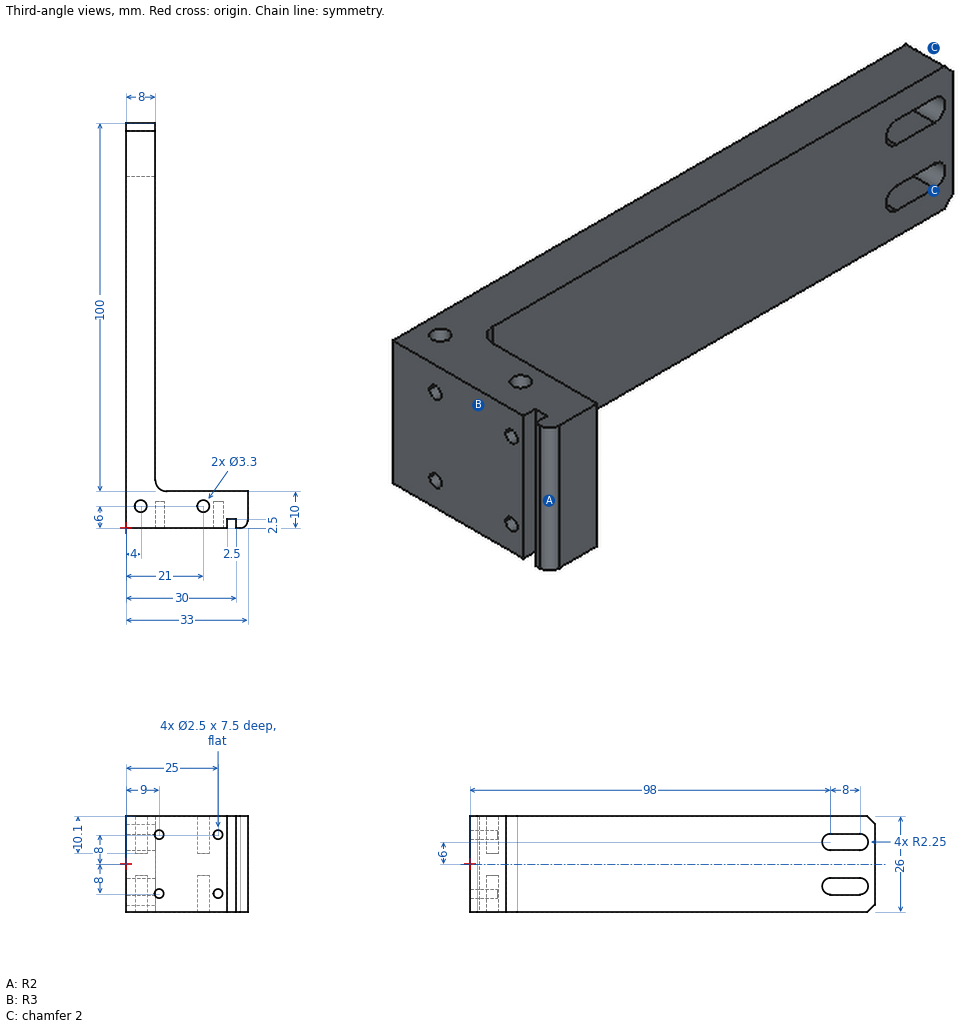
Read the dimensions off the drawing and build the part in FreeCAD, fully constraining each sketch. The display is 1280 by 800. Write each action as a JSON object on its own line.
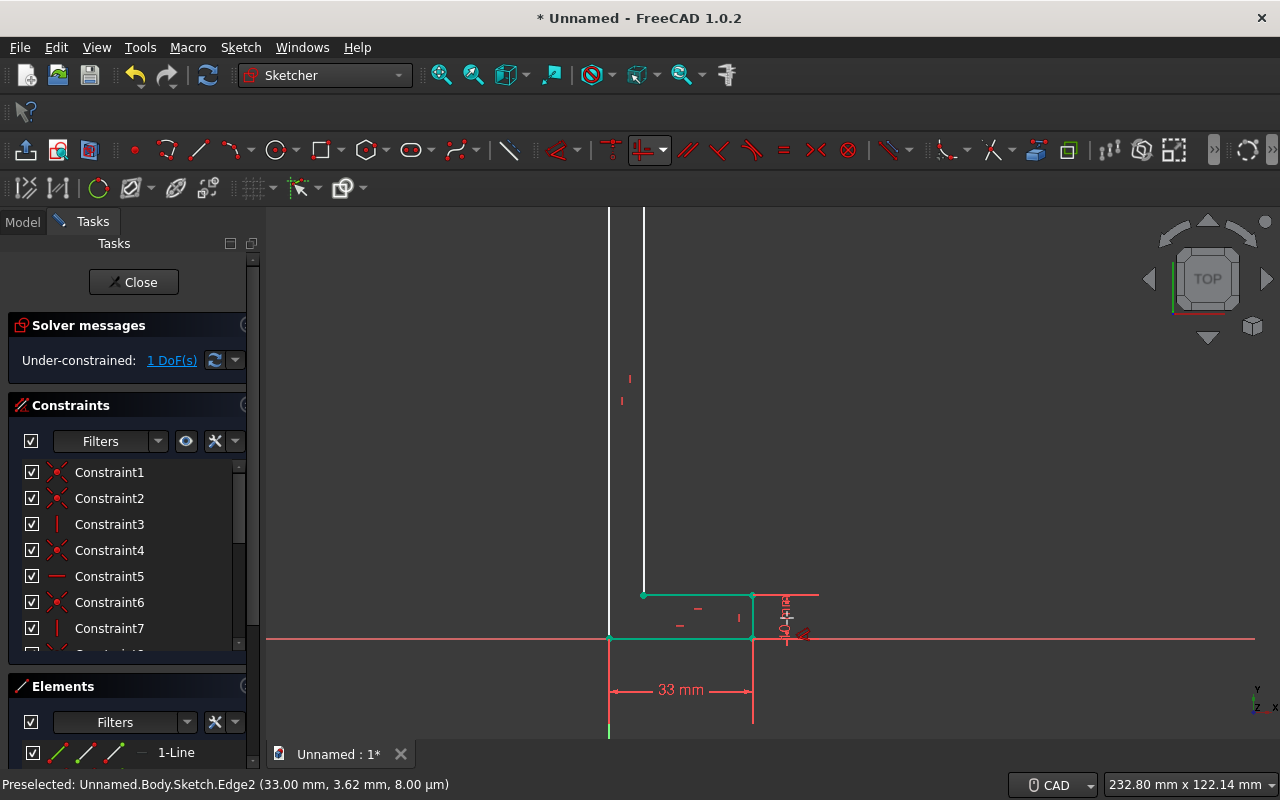
{"action": "left_click", "coordinate": [644, 465]}
{"action": "left_click", "coordinate": [678, 415]}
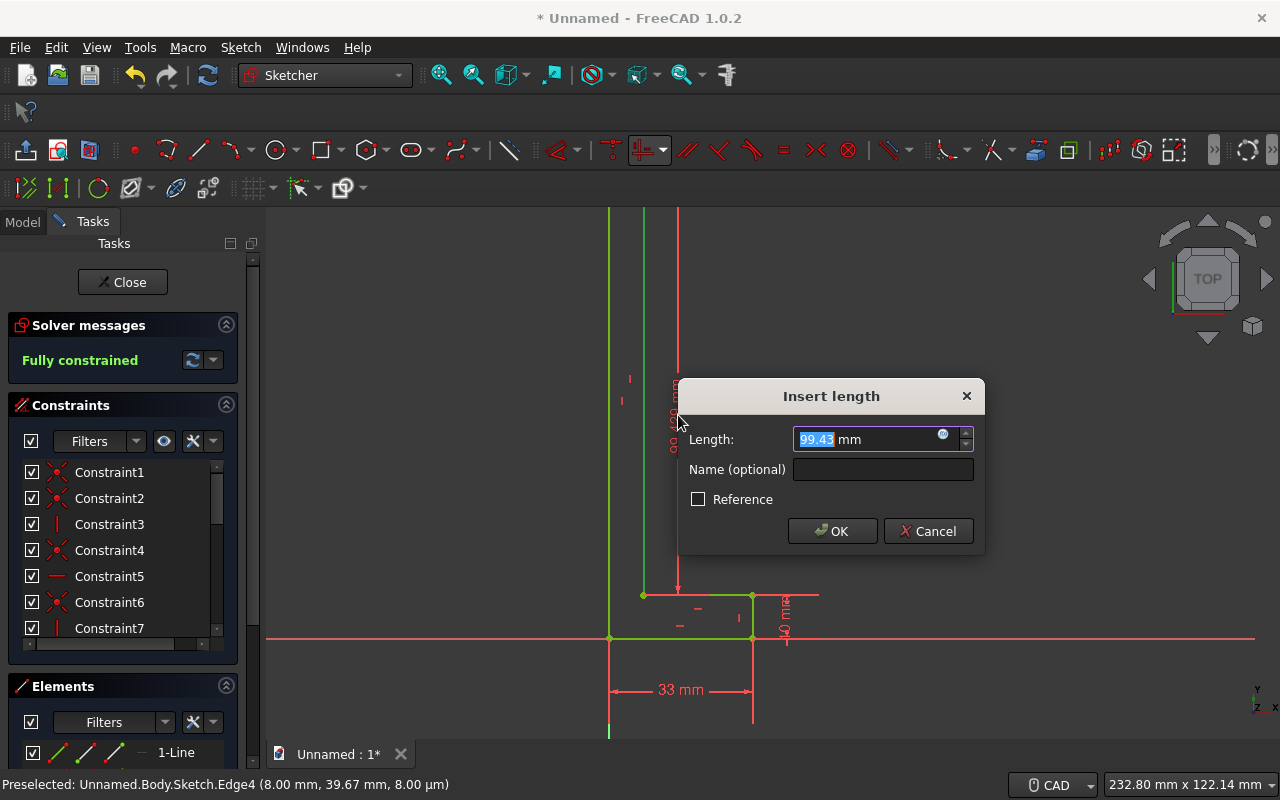
{"action": "type", "text": "100"}
{"action": "key", "text": "Return"}
{"action": "key", "text": "Escape"}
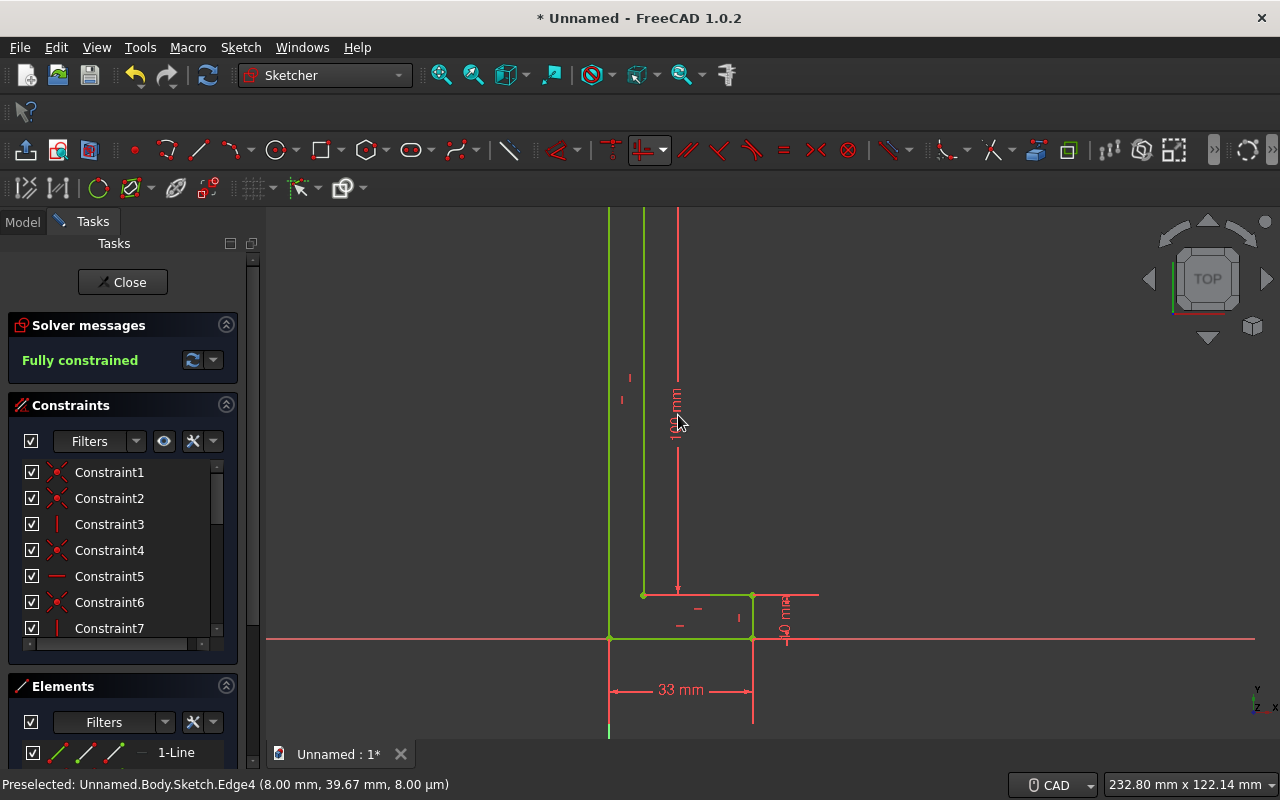
{"action": "left_click", "coordinate": [123, 282]}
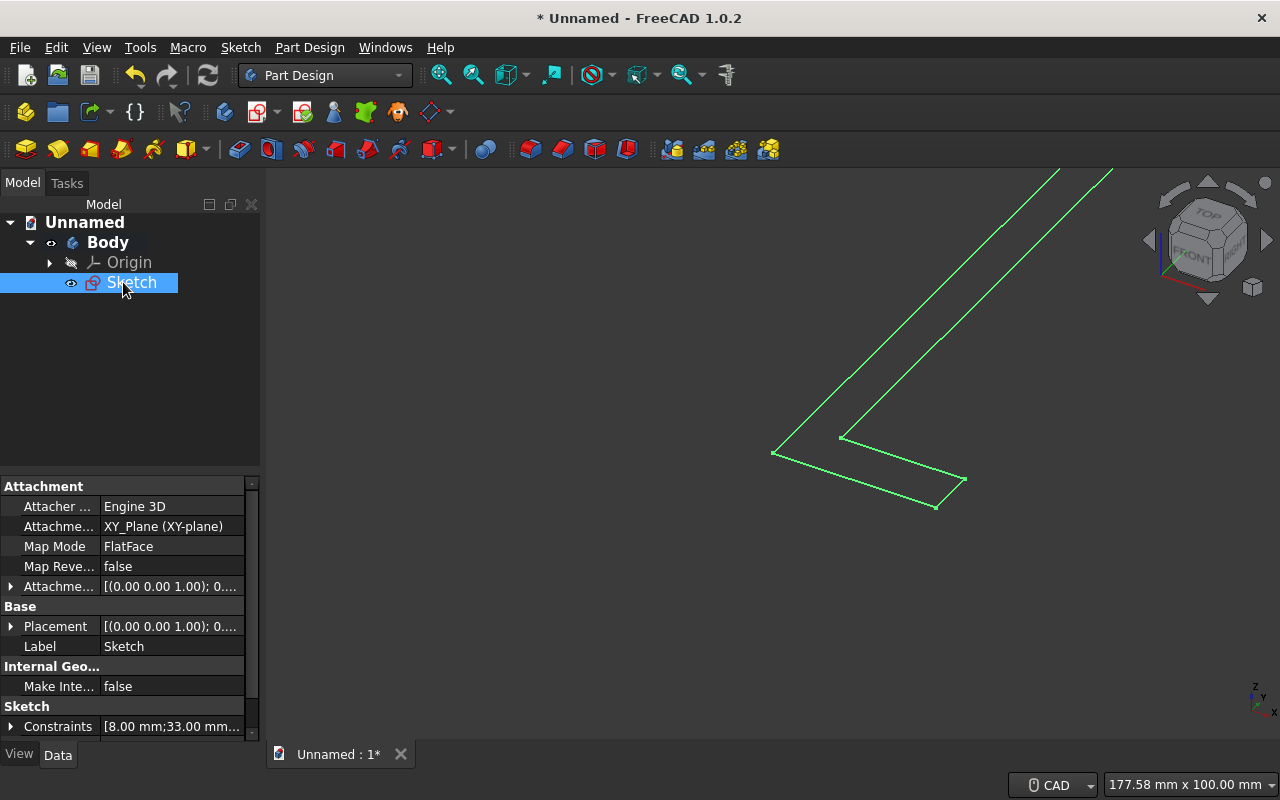
{"action": "left_click", "coordinate": [26, 150]}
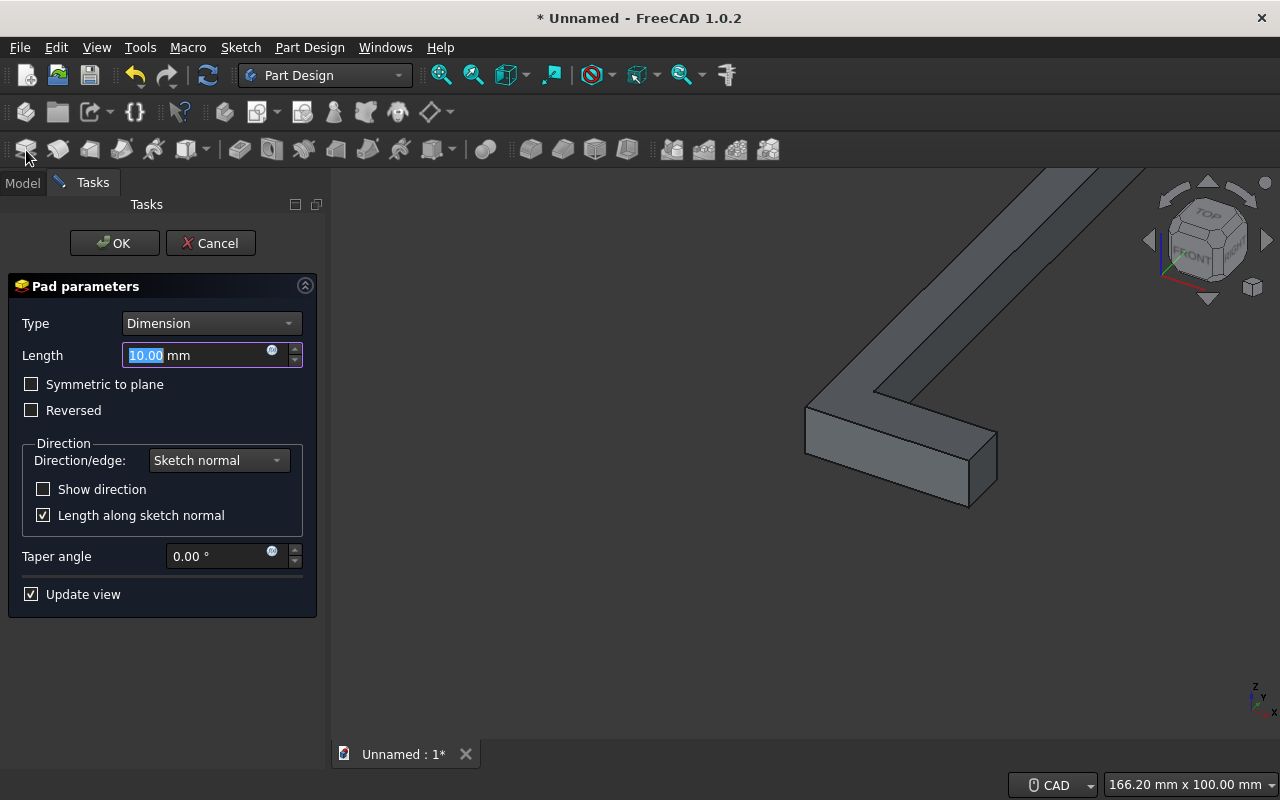
{"action": "type", "text": "26"}
{"action": "key", "text": "Tab"}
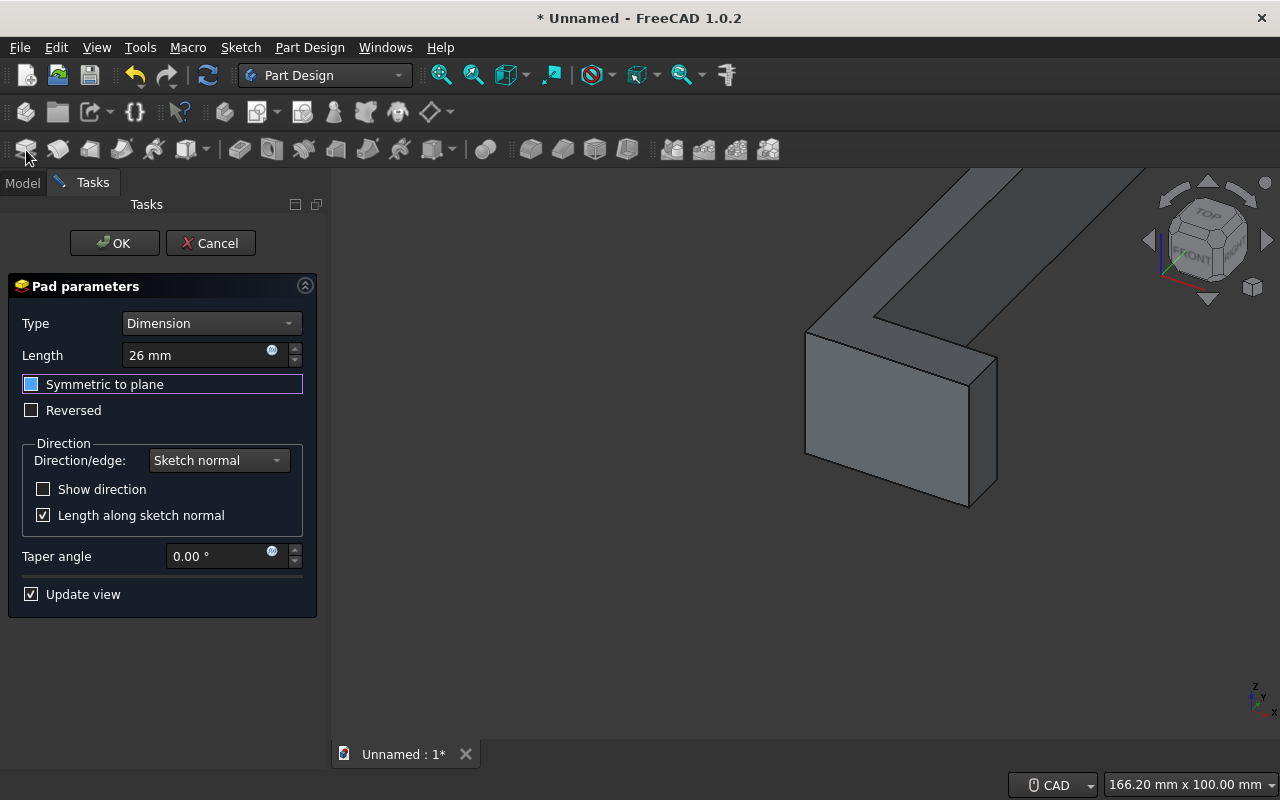
{"action": "left_click", "coordinate": [30, 384]}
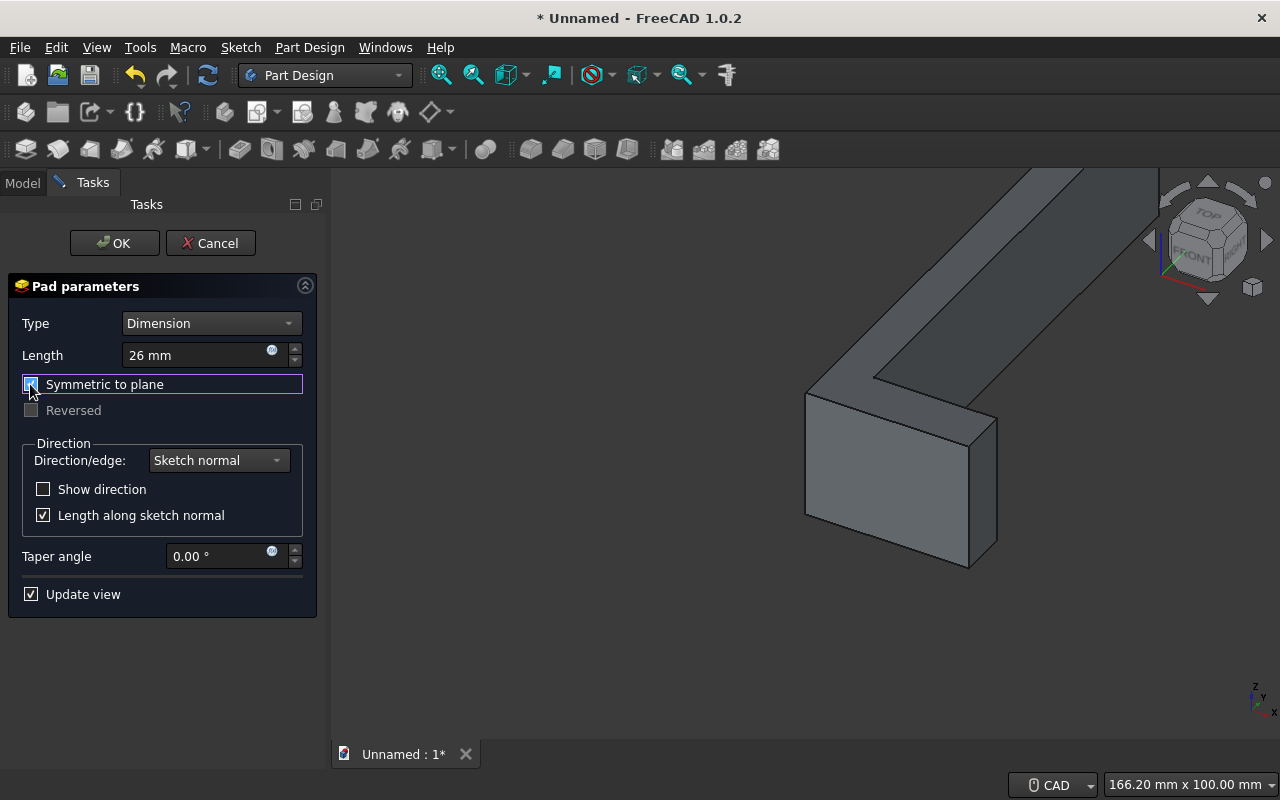
{"action": "left_click", "coordinate": [115, 243]}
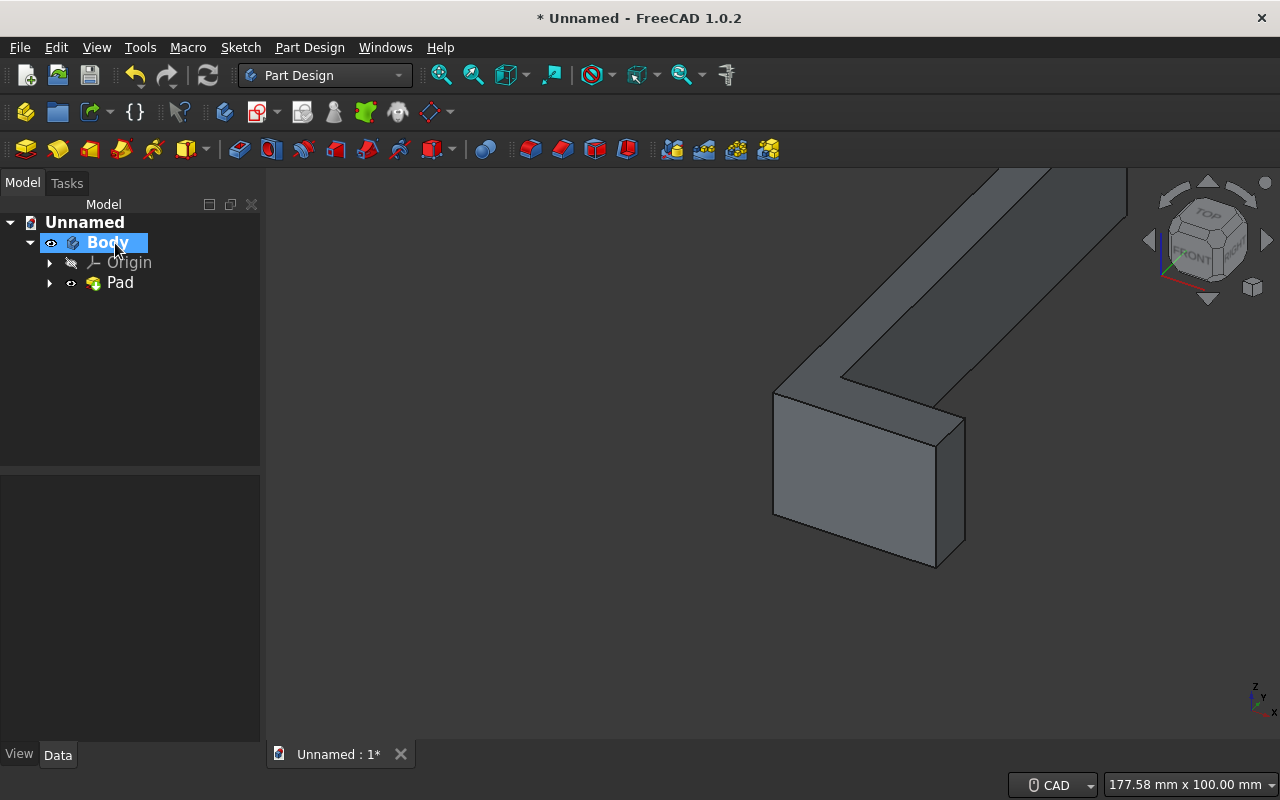
{"action": "left_click", "coordinate": [442, 76]}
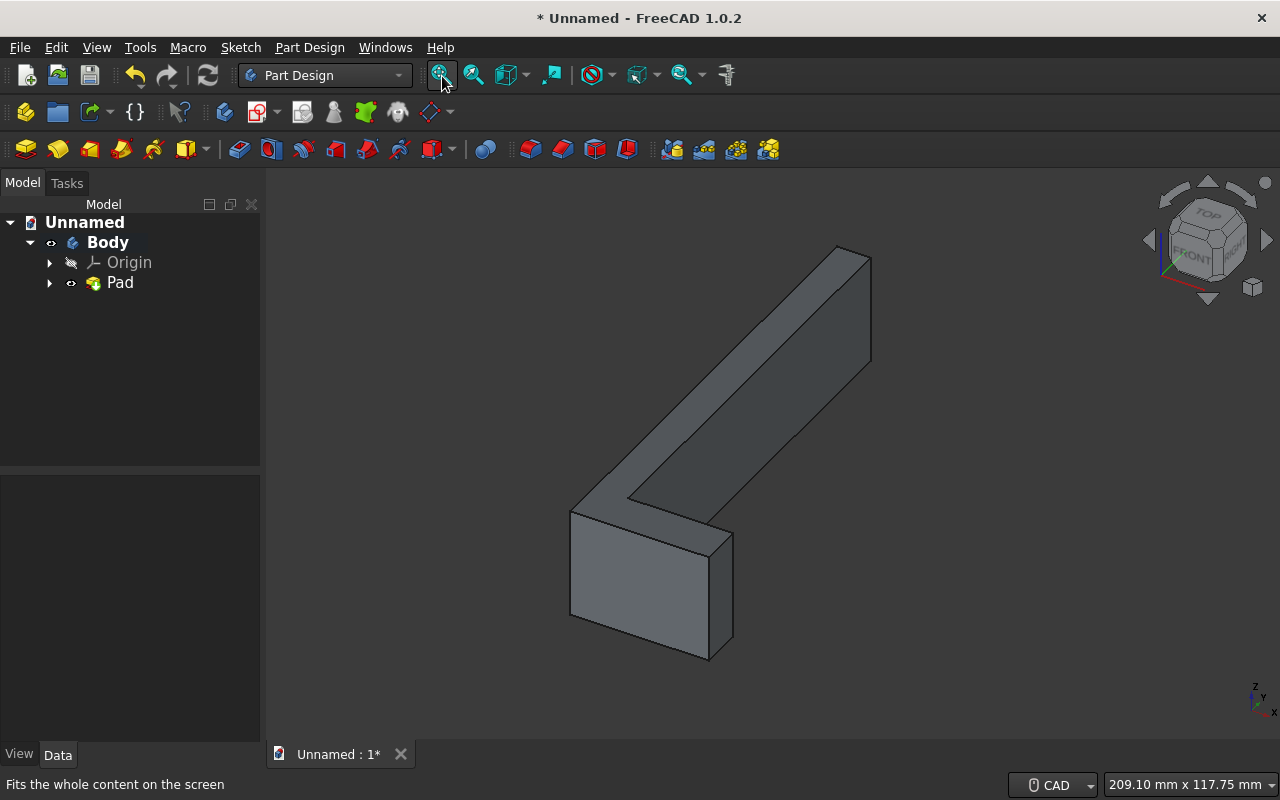
{"action": "left_click", "coordinate": [828, 268]}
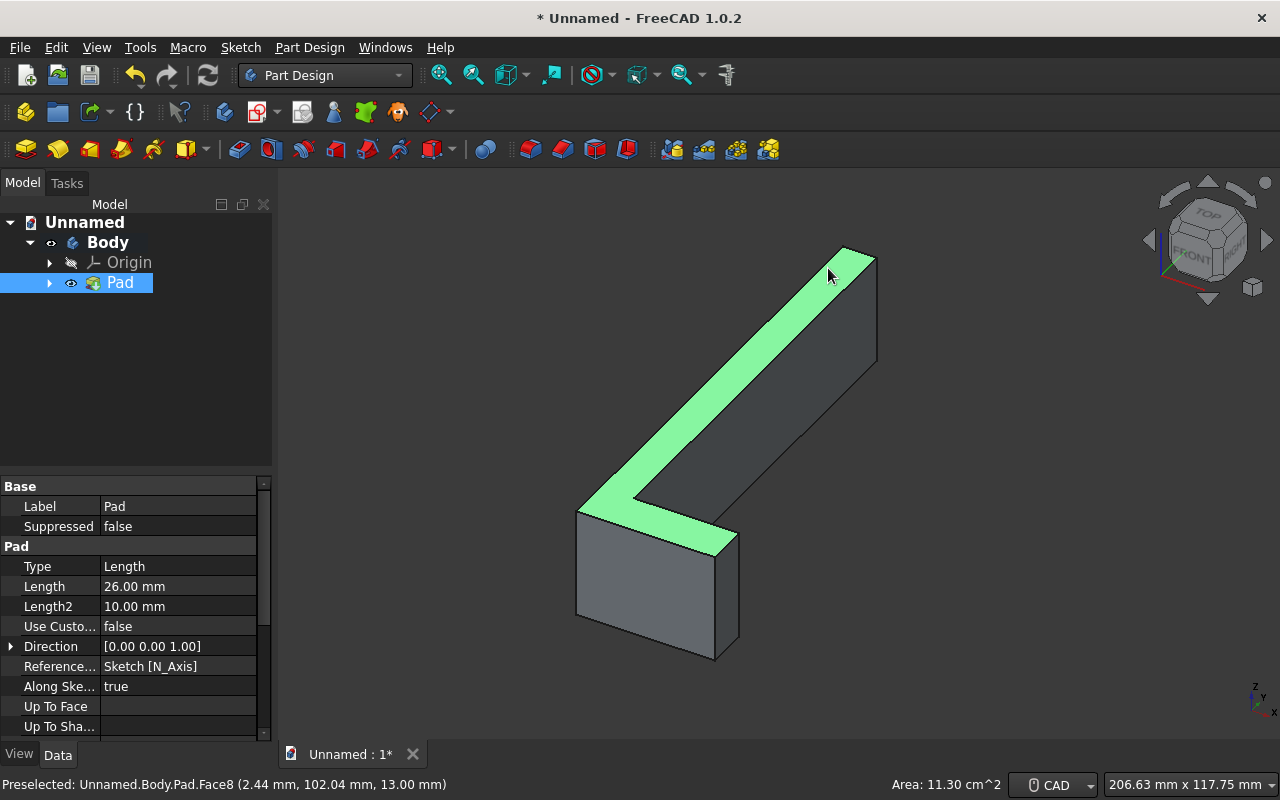
{"action": "left_click", "coordinate": [258, 112]}